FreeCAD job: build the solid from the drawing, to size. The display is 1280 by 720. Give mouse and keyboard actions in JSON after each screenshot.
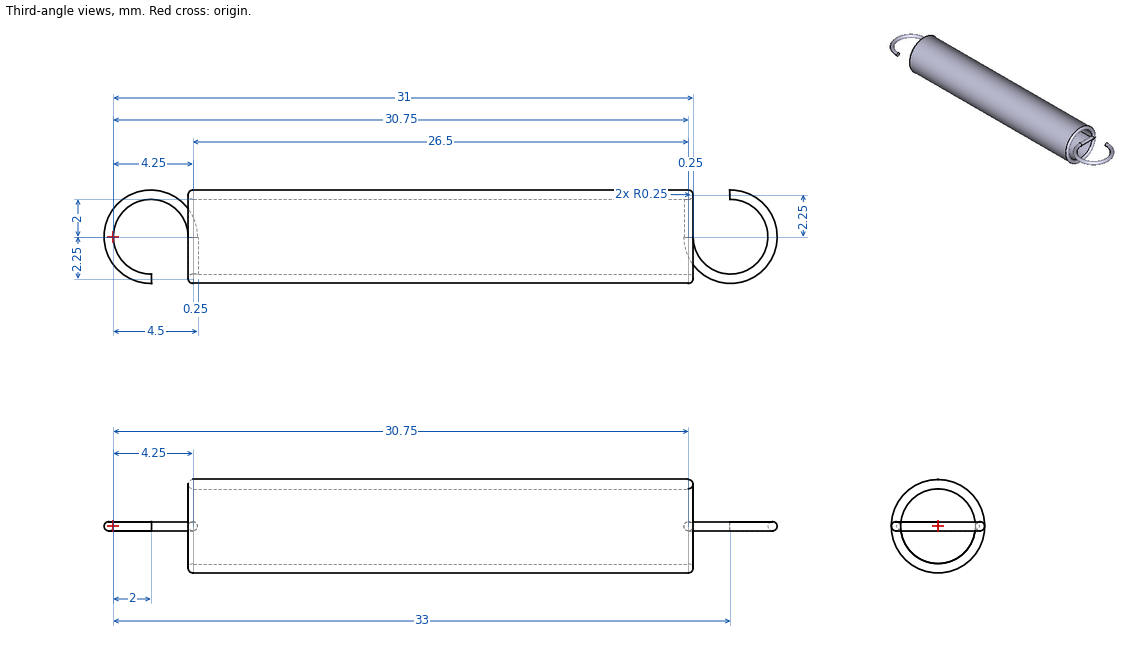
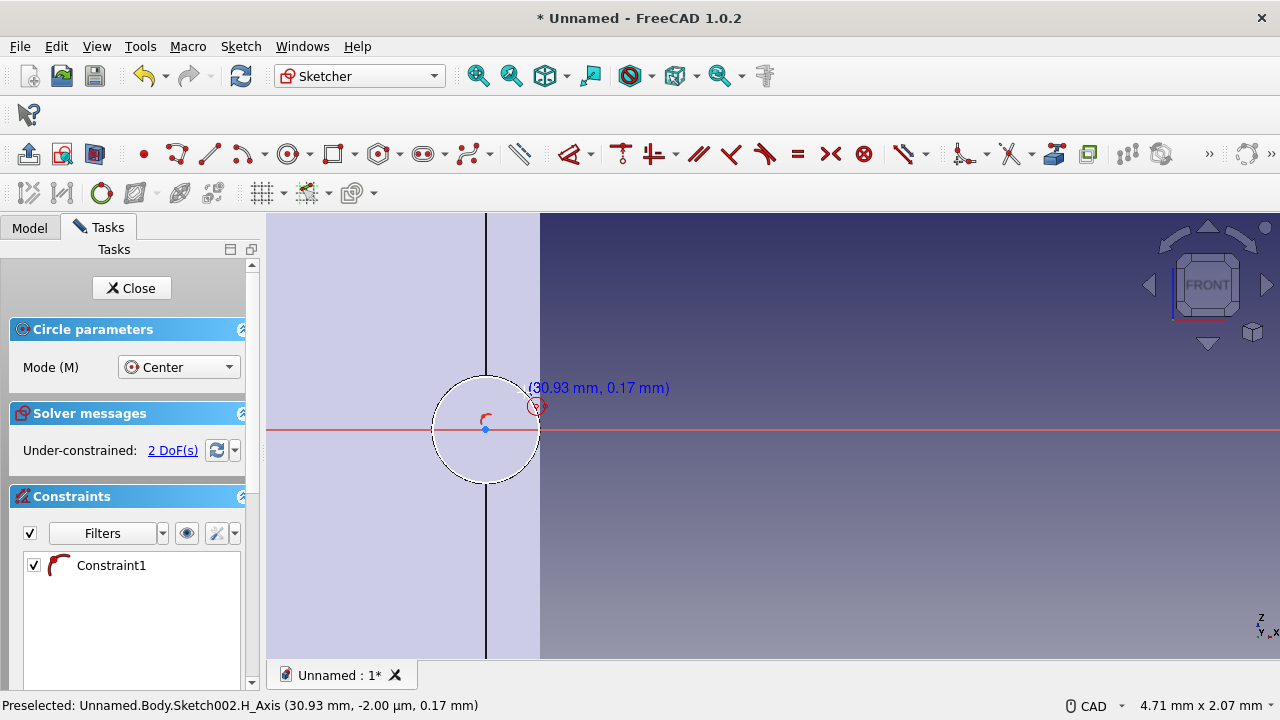
{"action": "left_click", "coordinate": [210, 154]}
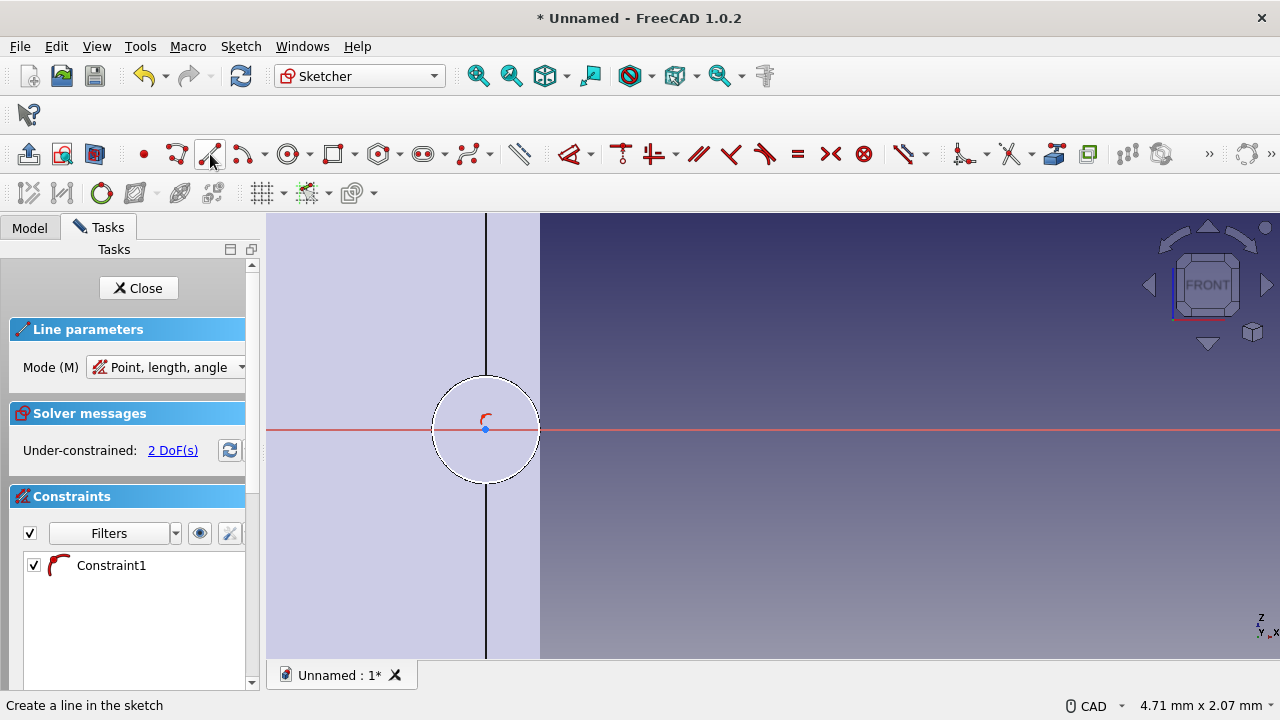
{"action": "left_click", "coordinate": [970, 494]}
{"action": "left_click", "coordinate": [970, 365]}
{"action": "key", "text": "Escape"}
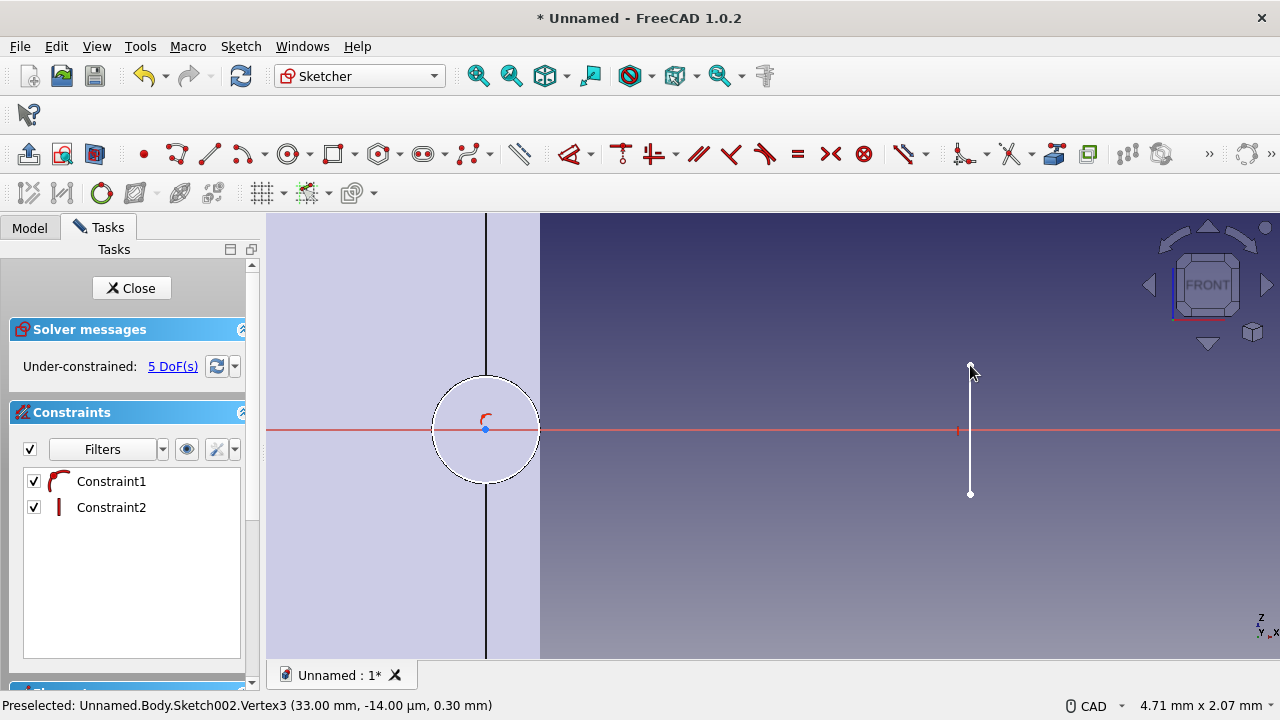
{"action": "left_click", "coordinate": [970, 456]}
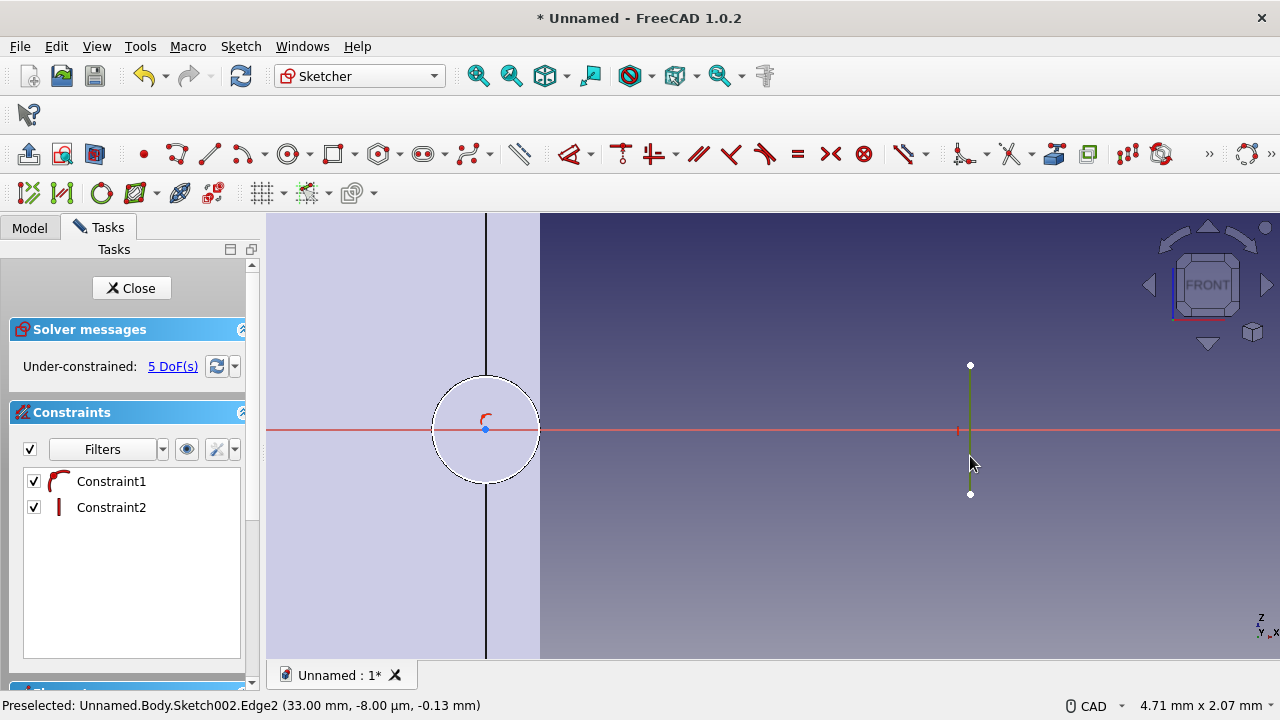
{"action": "key", "text": "g n"}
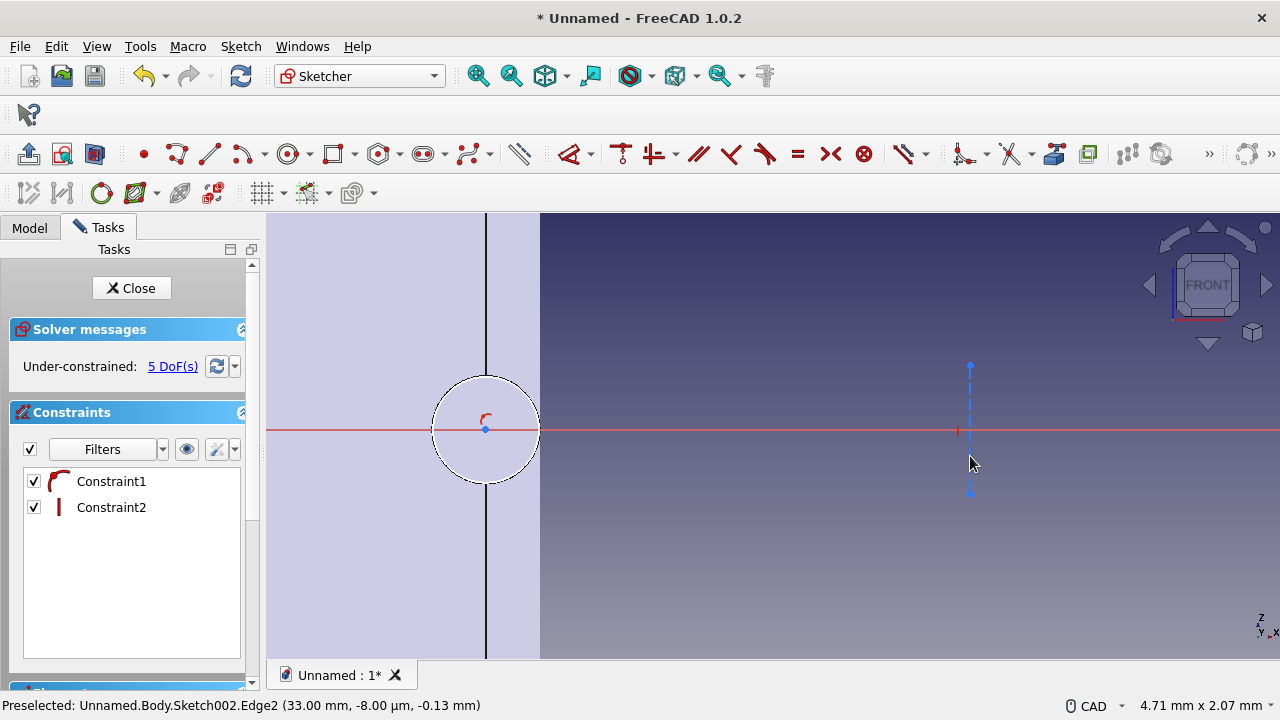
{"action": "key", "text": "d"}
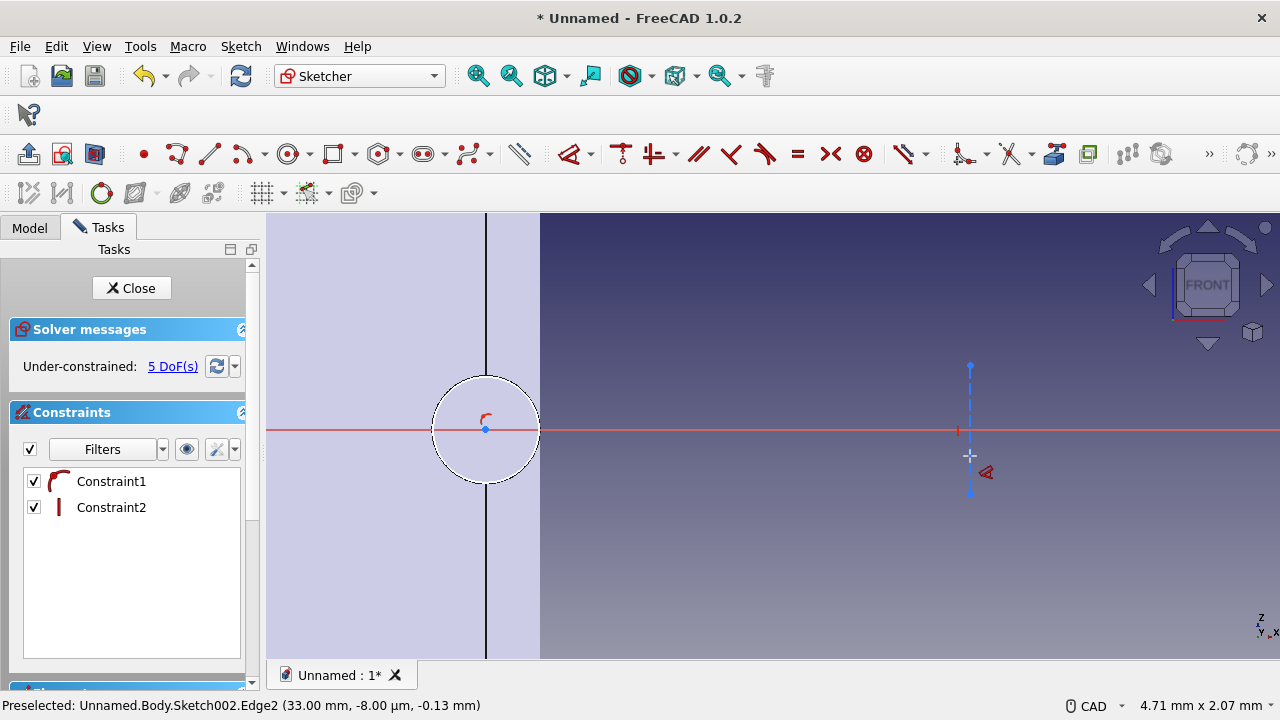
{"action": "left_click", "coordinate": [523, 392]}
{"action": "left_click", "coordinate": [545, 369]}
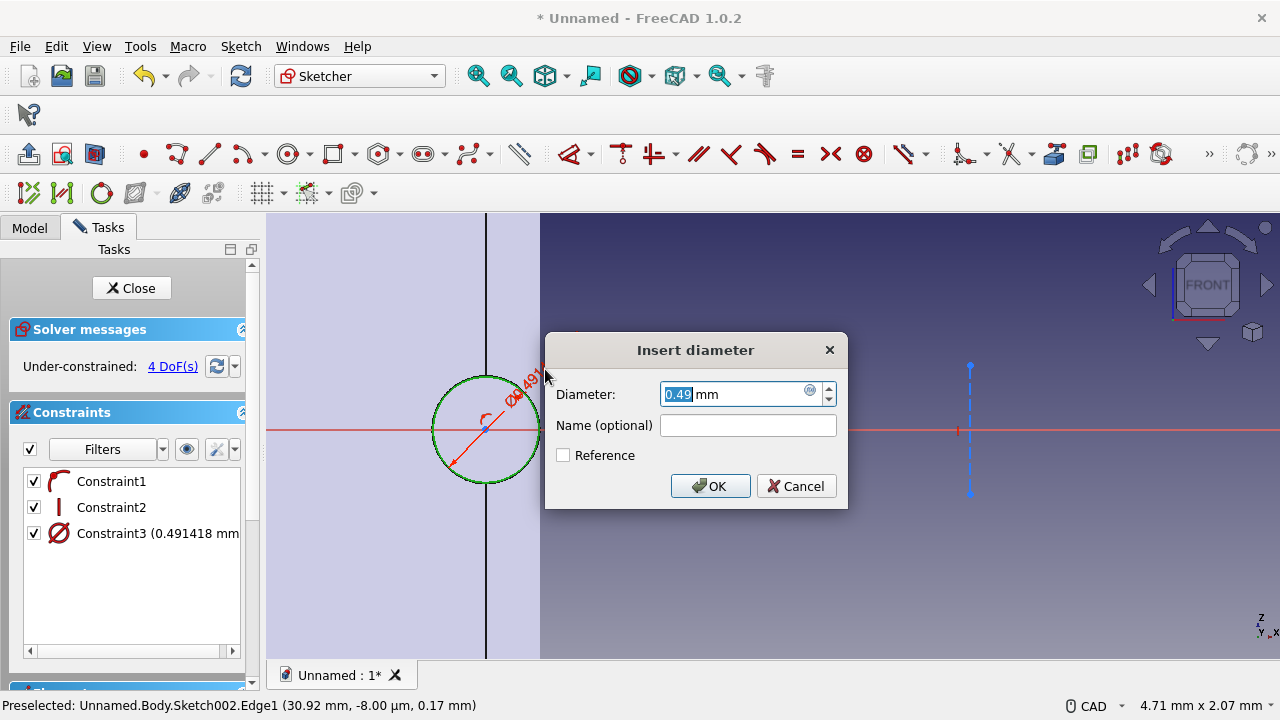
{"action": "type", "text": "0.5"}
{"action": "key", "text": "Return"}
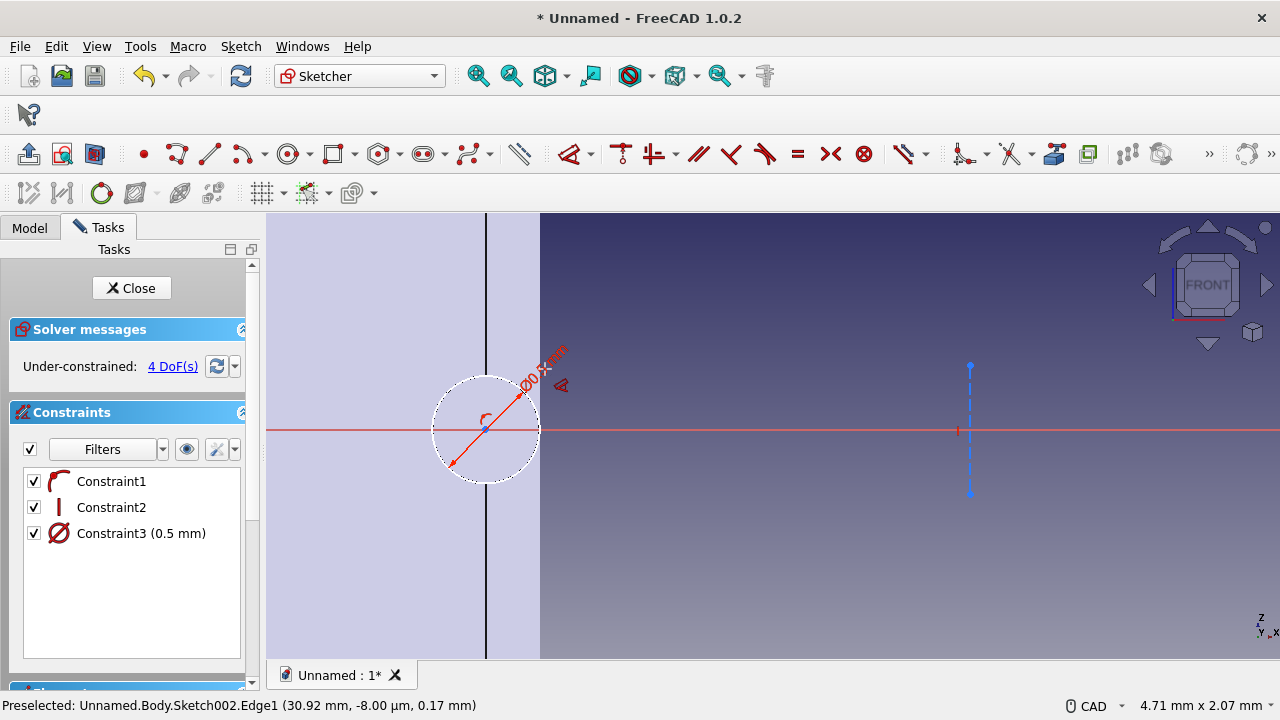
{"action": "left_click", "coordinate": [970, 495]}
{"action": "left_click", "coordinate": [632, 529]}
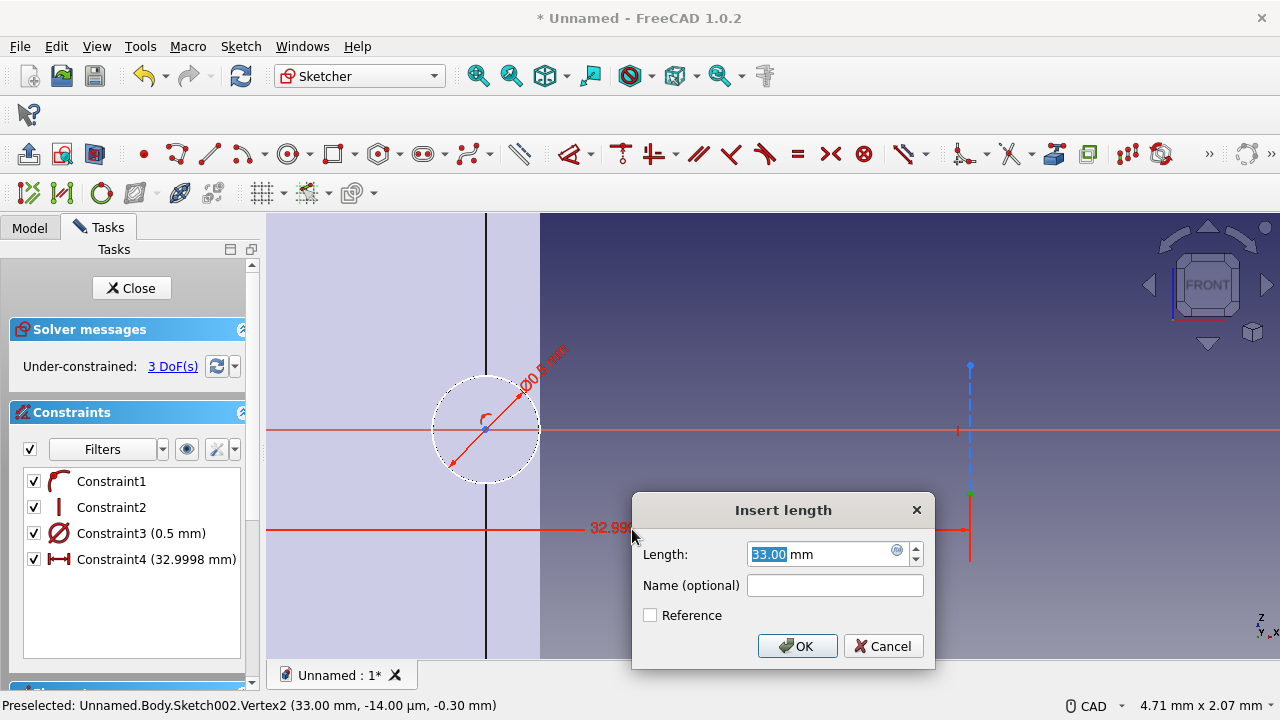
{"action": "type", "text": "33"}
{"action": "key", "text": "Return"}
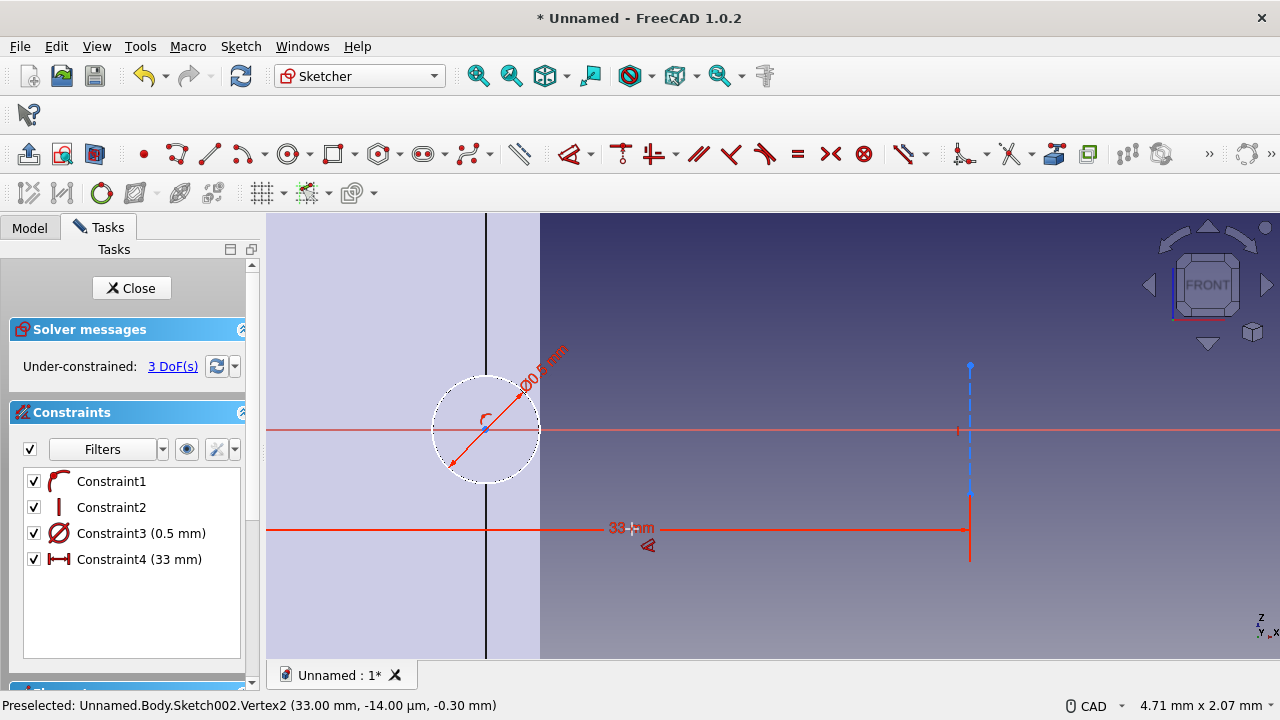
{"action": "left_click", "coordinate": [486, 430]}
{"action": "left_click", "coordinate": [390, 464]}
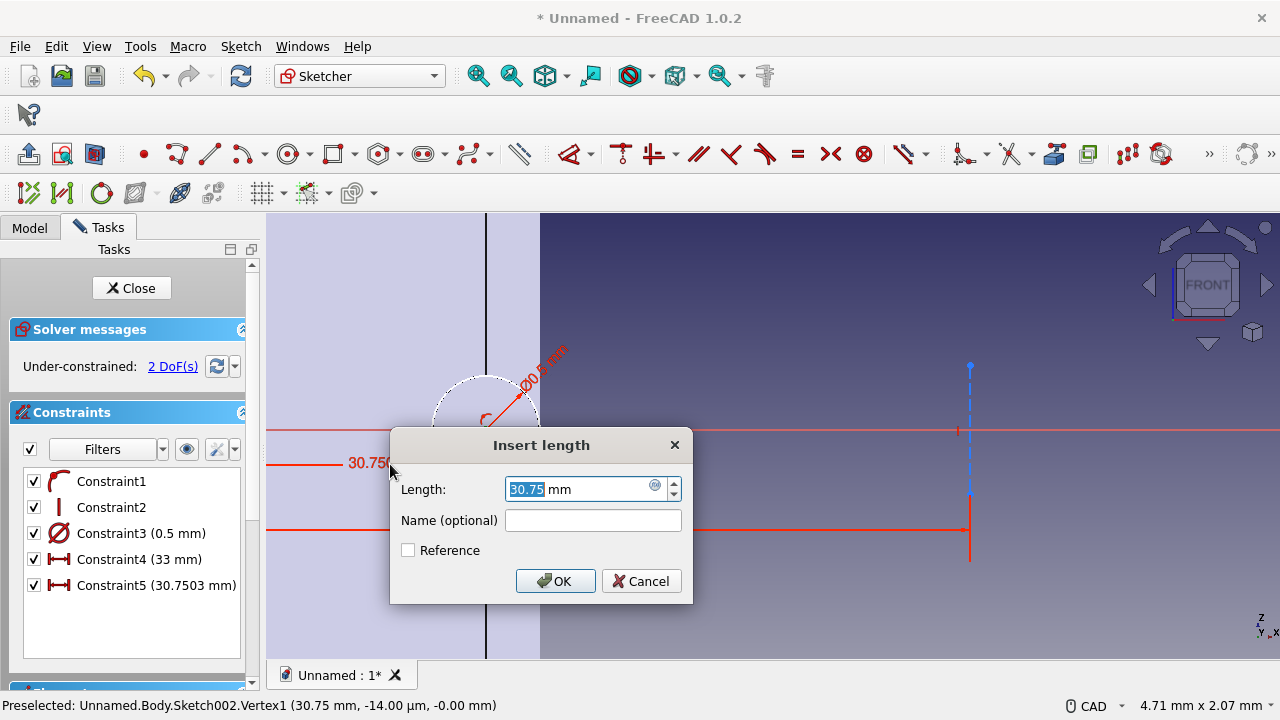
{"action": "type", "text": "30.75"}
{"action": "key", "text": "Return"}
{"action": "key", "text": "Escape"}